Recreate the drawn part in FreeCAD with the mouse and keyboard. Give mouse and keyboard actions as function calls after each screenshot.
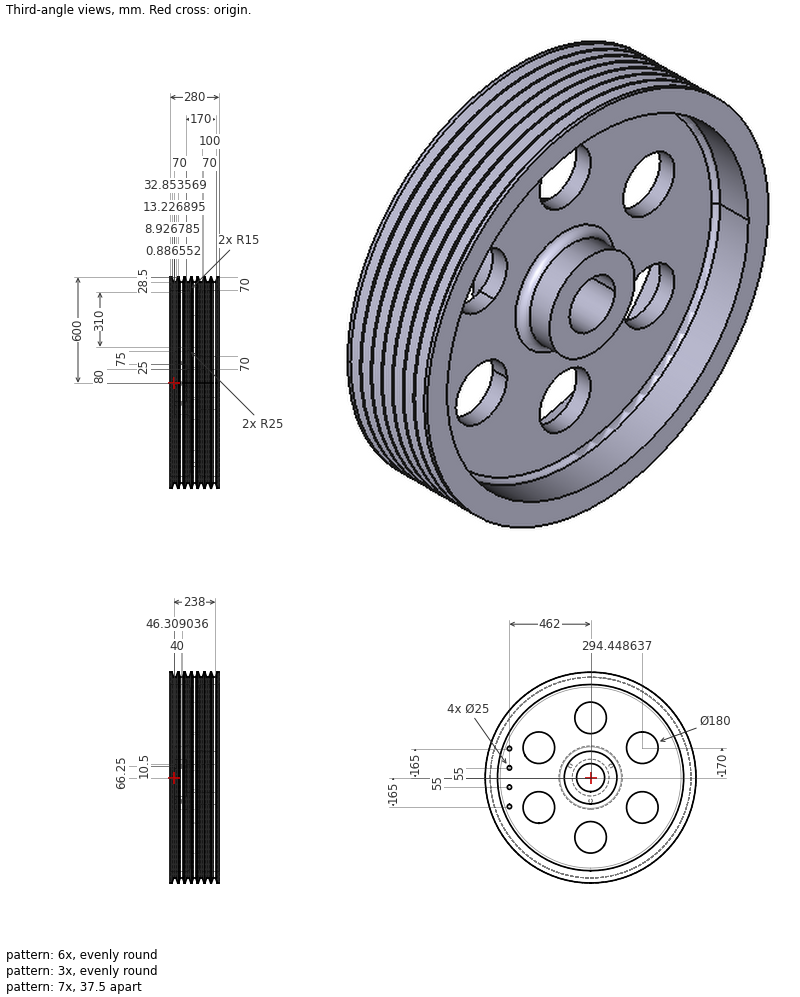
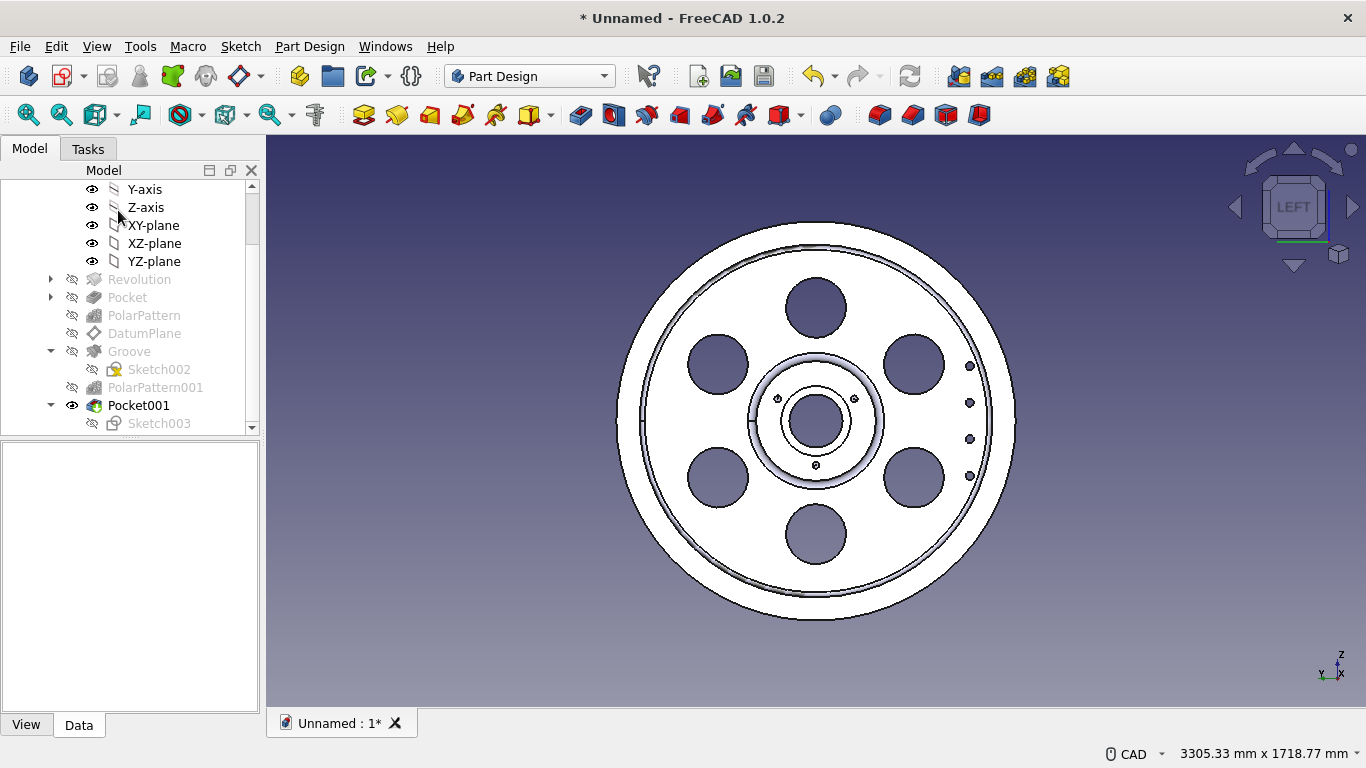
click(62, 76)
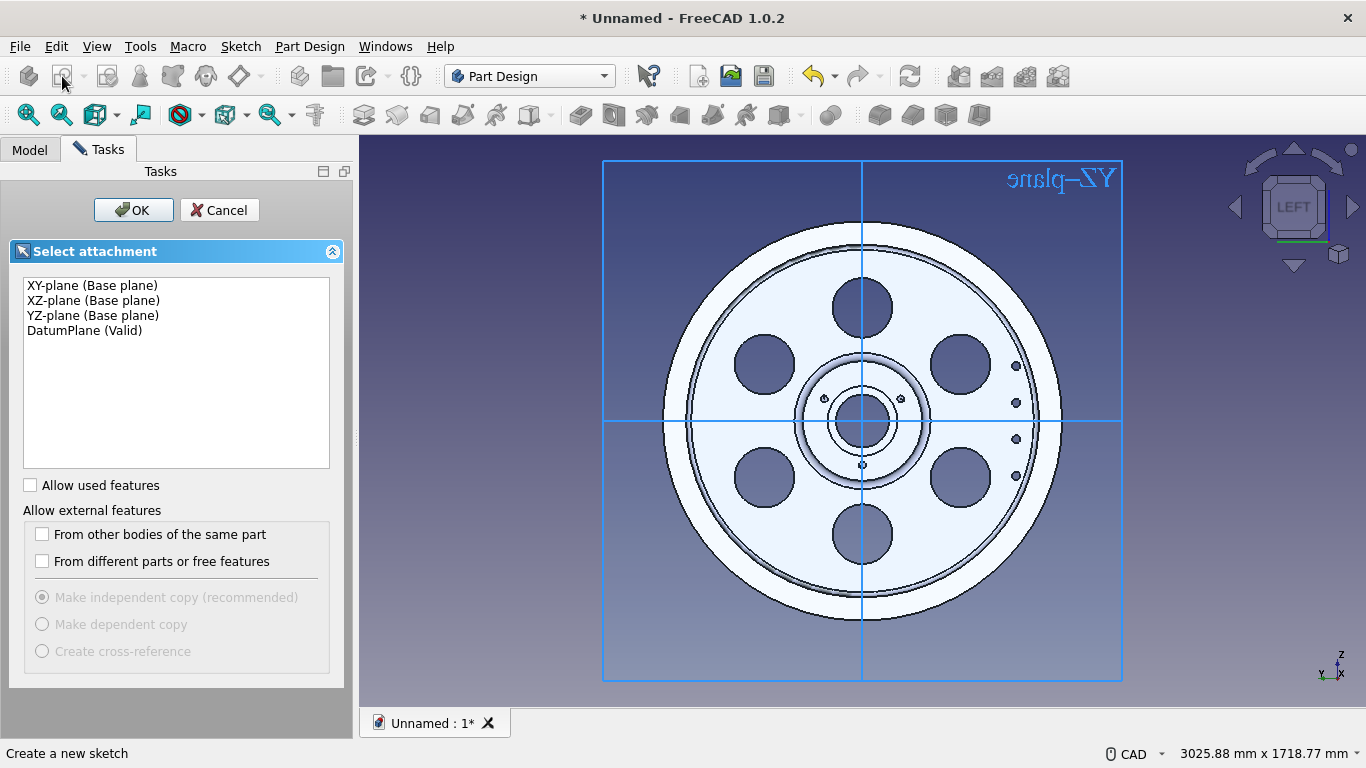
click(84, 286)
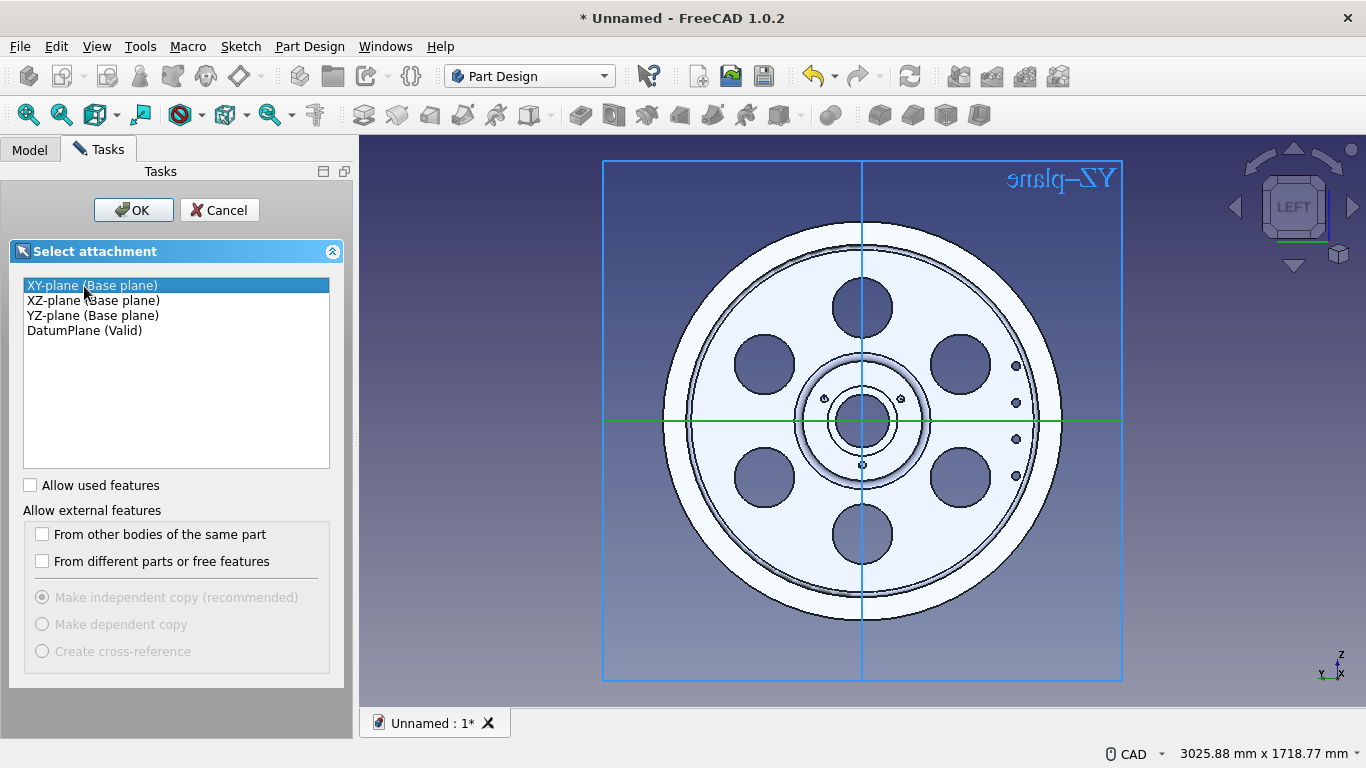
click(134, 210)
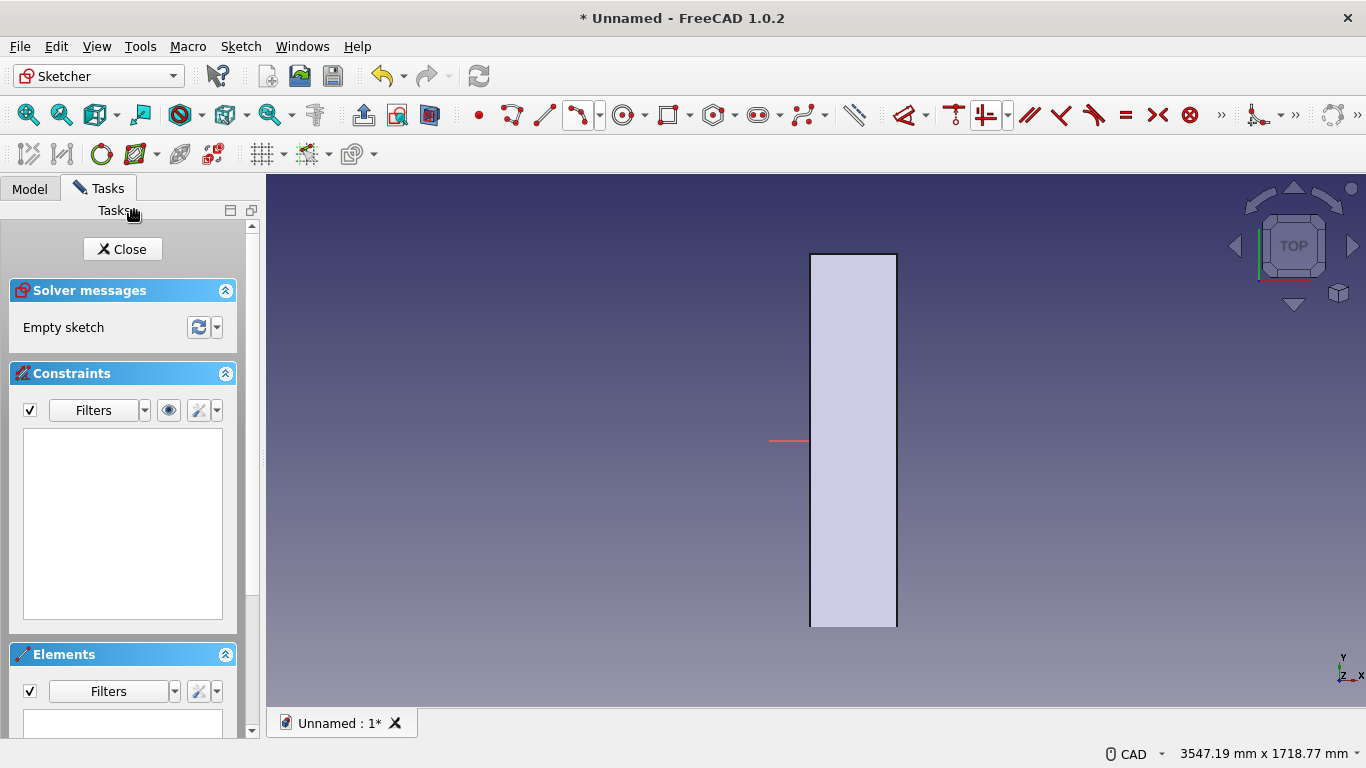
click(430, 116)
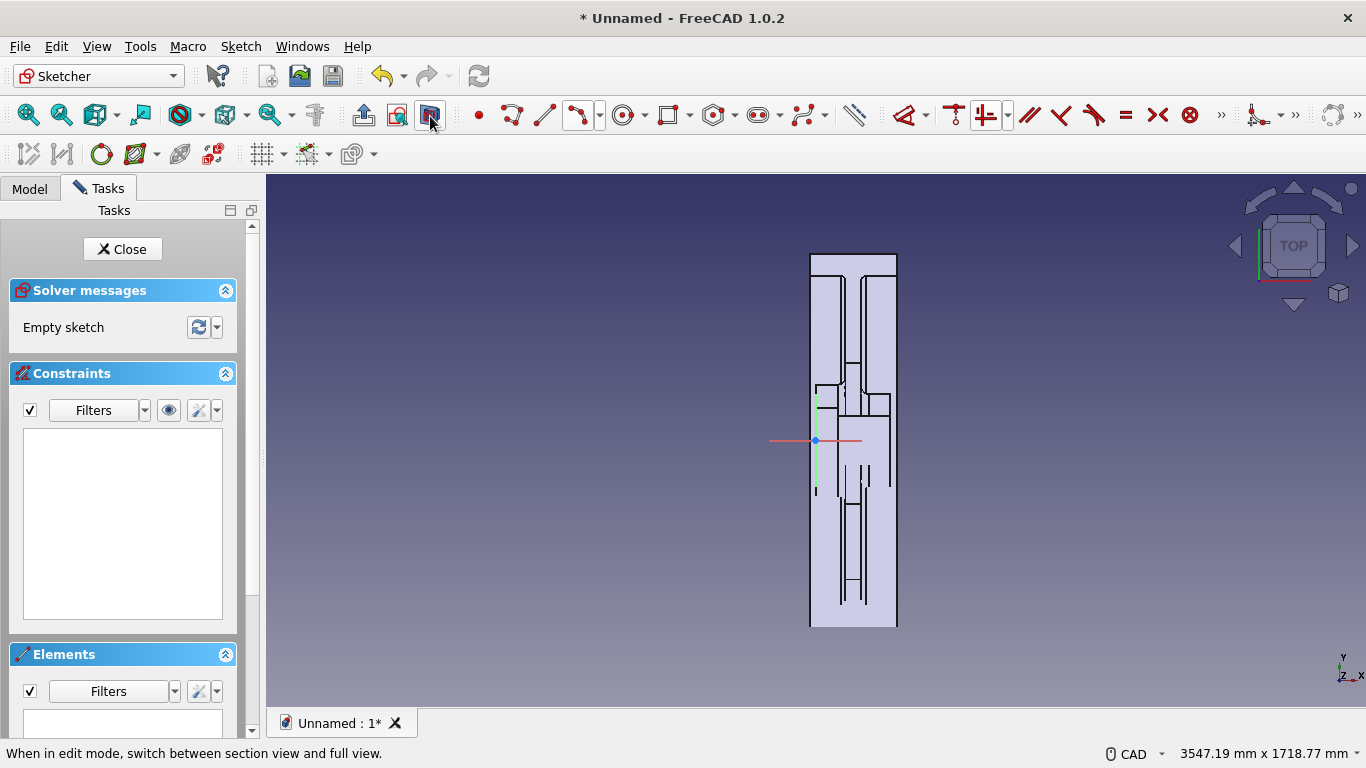
scroll(822, 249, up, 15)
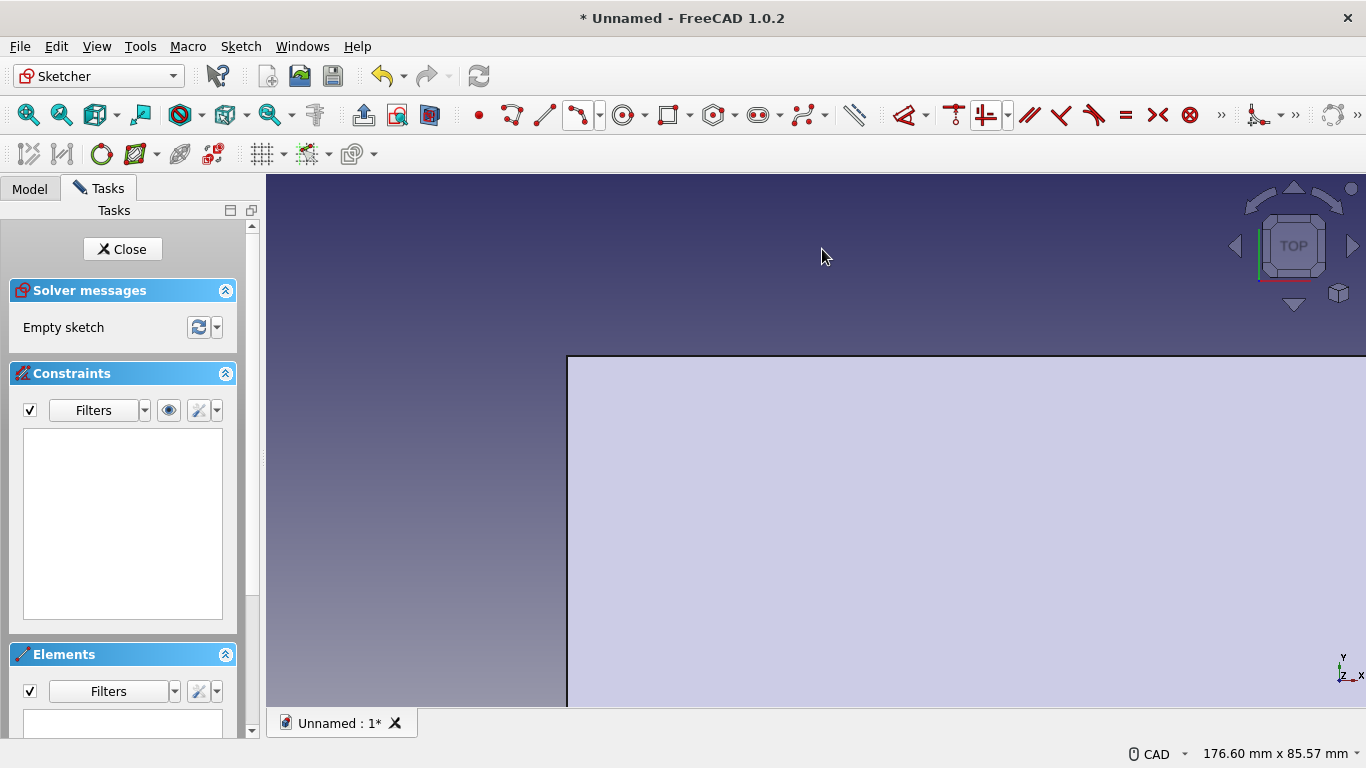
scroll(728, 449, up, 3)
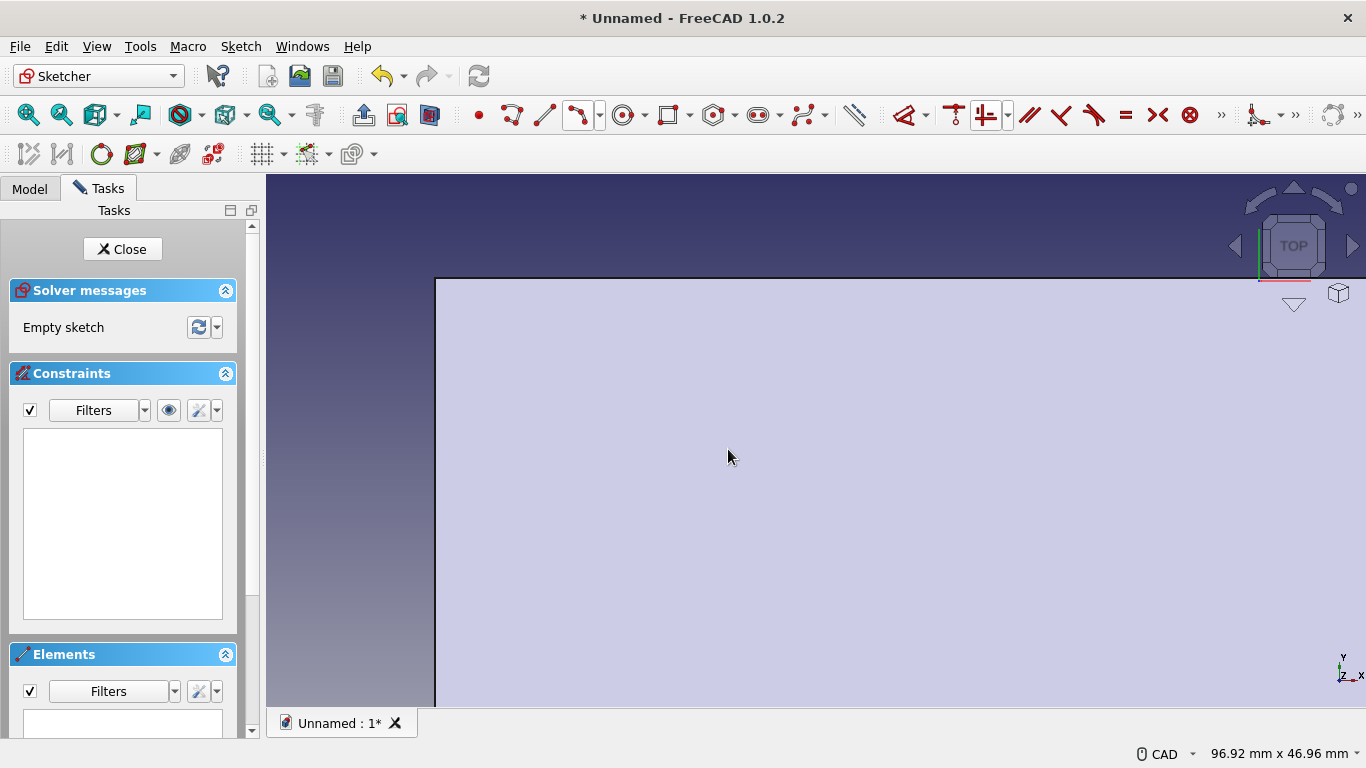
click(512, 116)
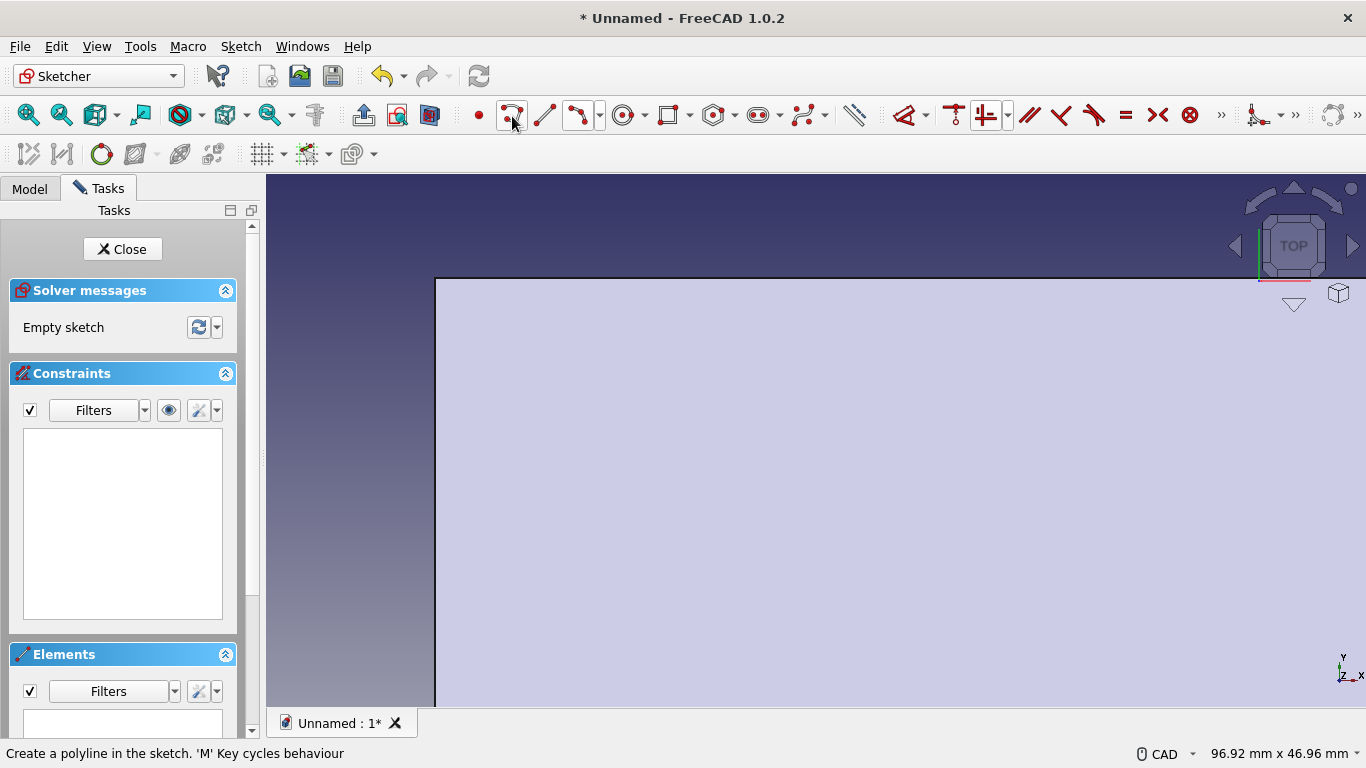
scroll(672, 602, up, 3)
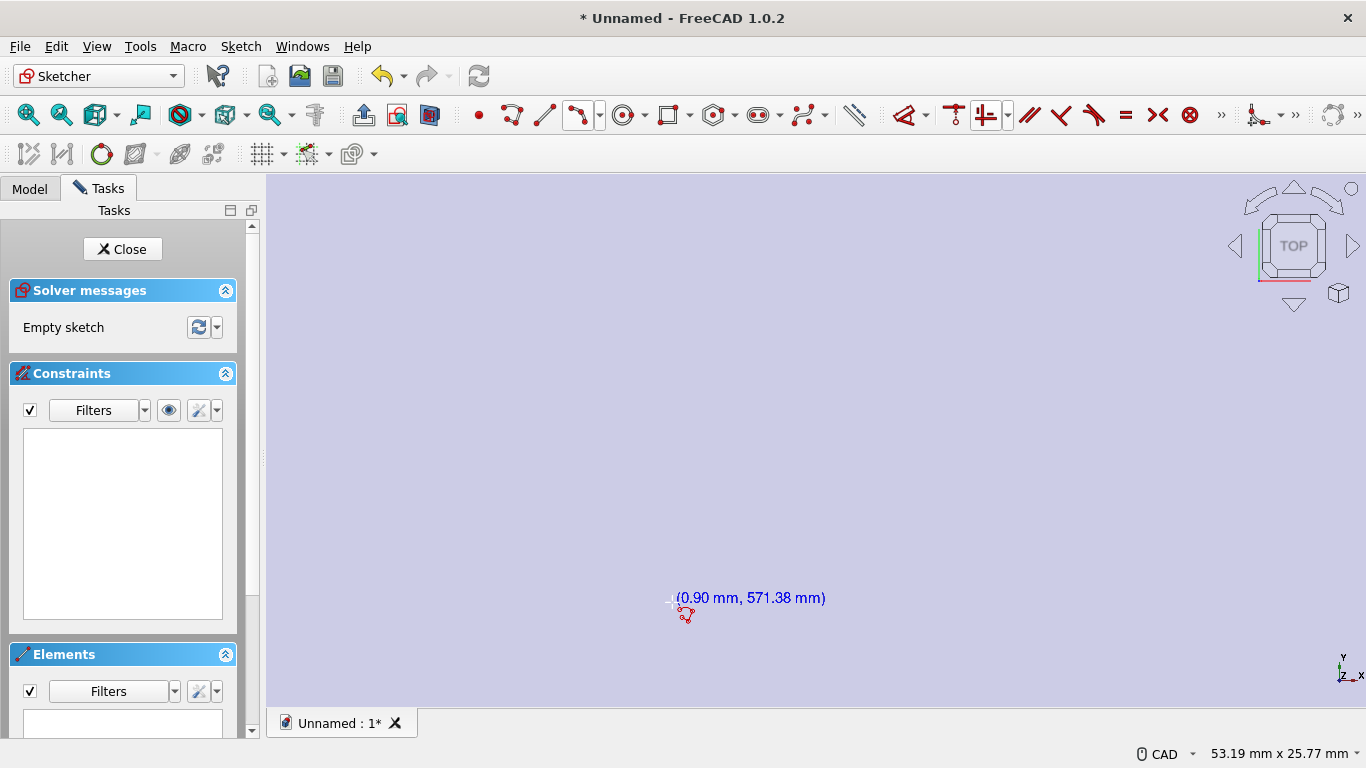
click(671, 601)
click(945, 601)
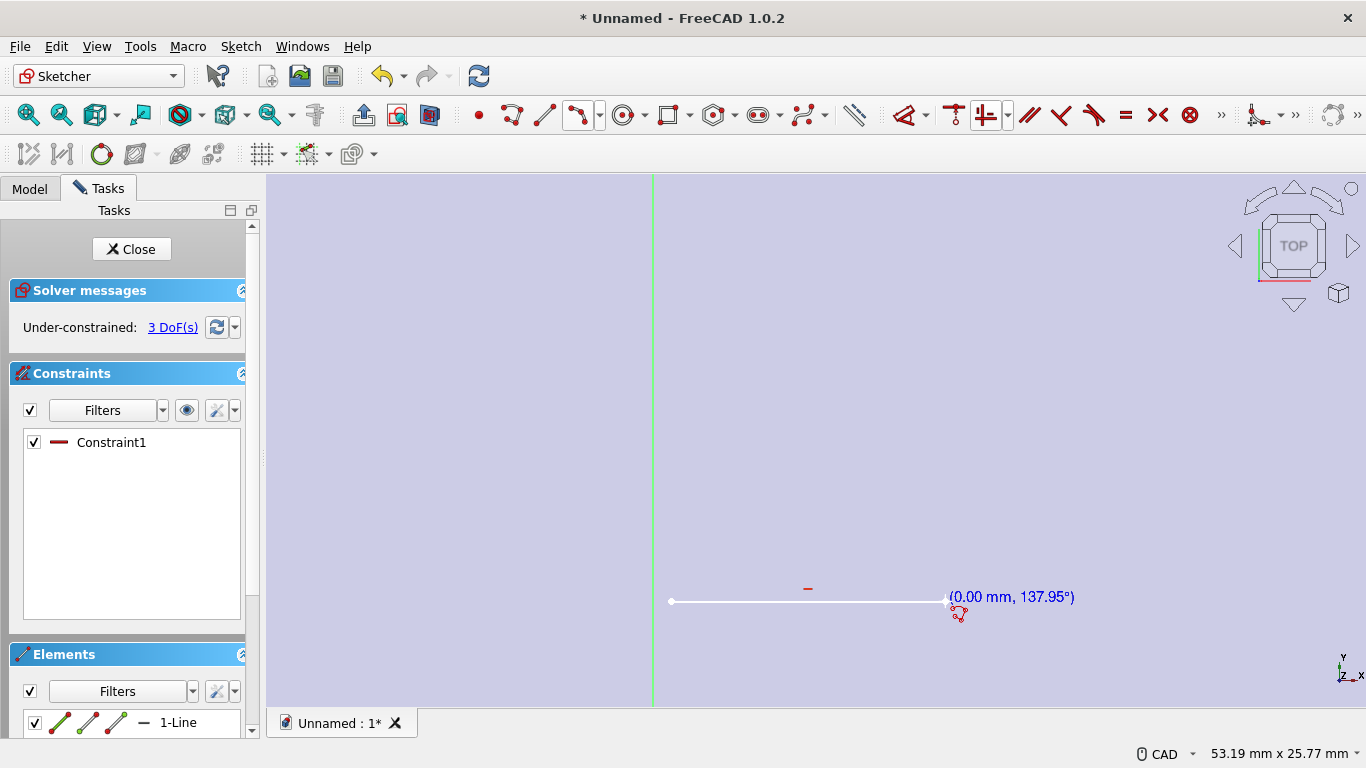
scroll(674, 604, down, 3)